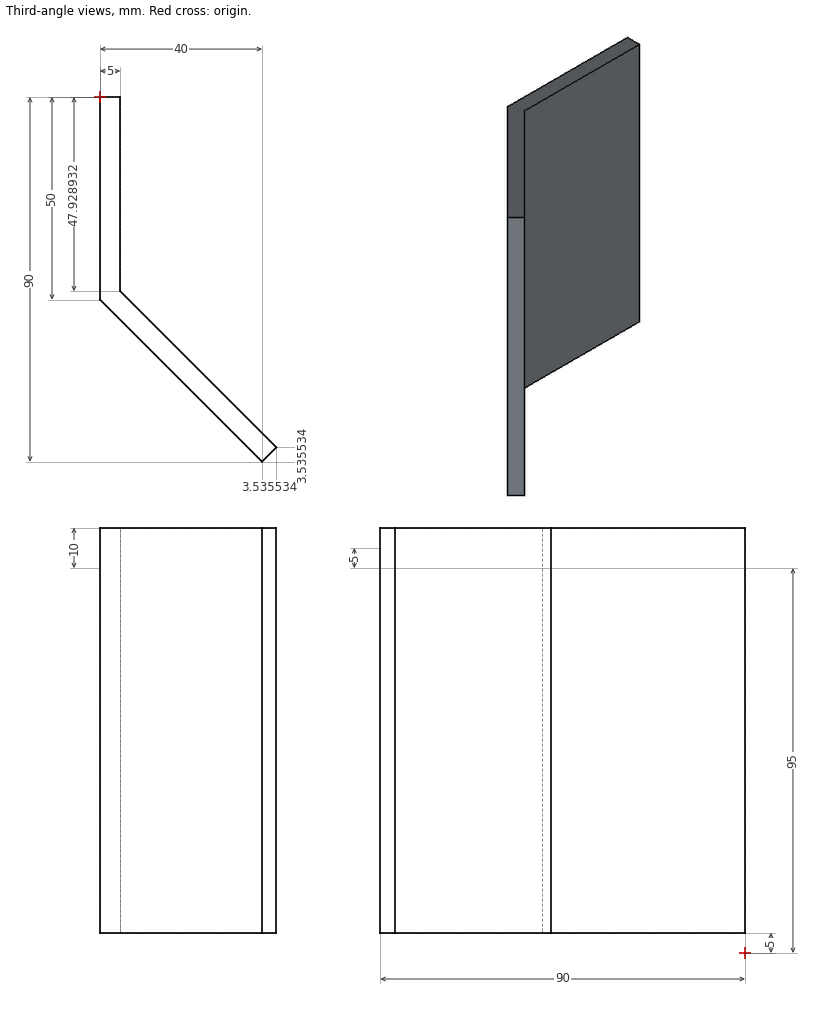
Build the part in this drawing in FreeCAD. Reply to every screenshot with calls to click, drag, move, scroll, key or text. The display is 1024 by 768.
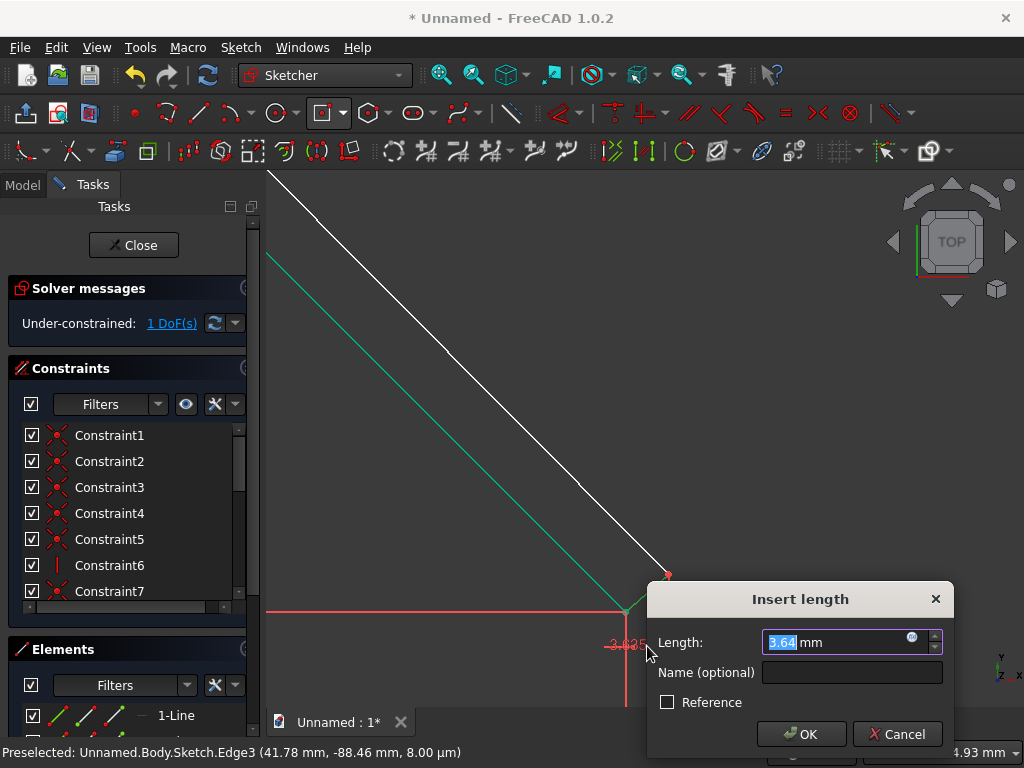
text(3.535534)
key(Return)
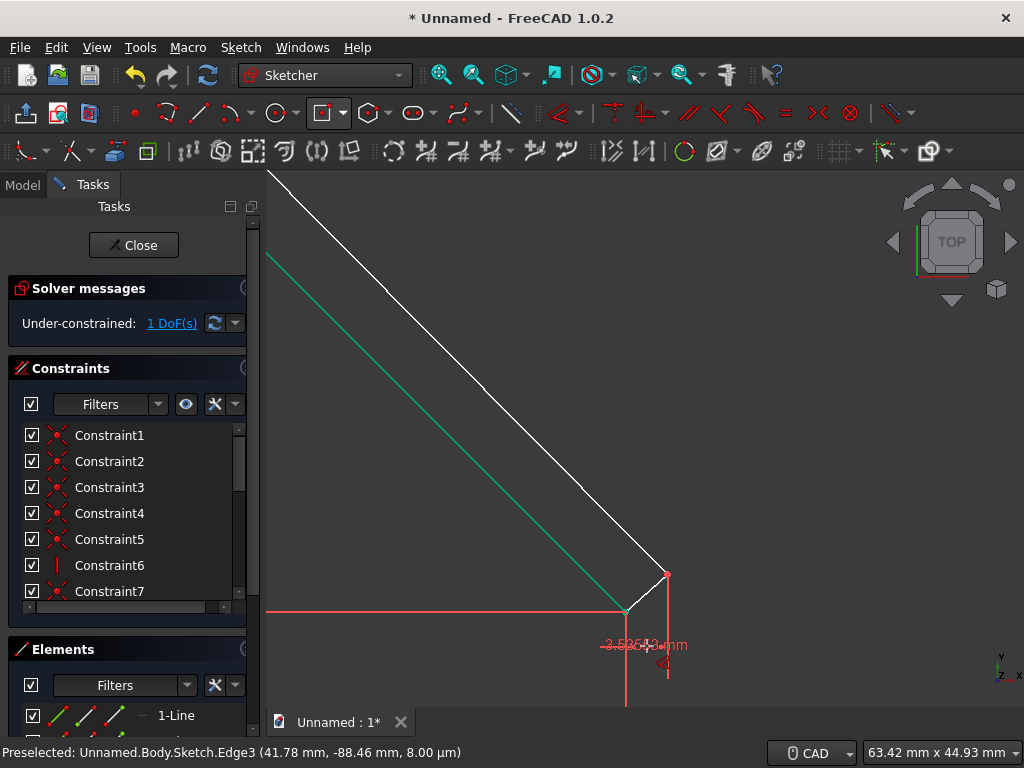
click(638, 601)
click(702, 593)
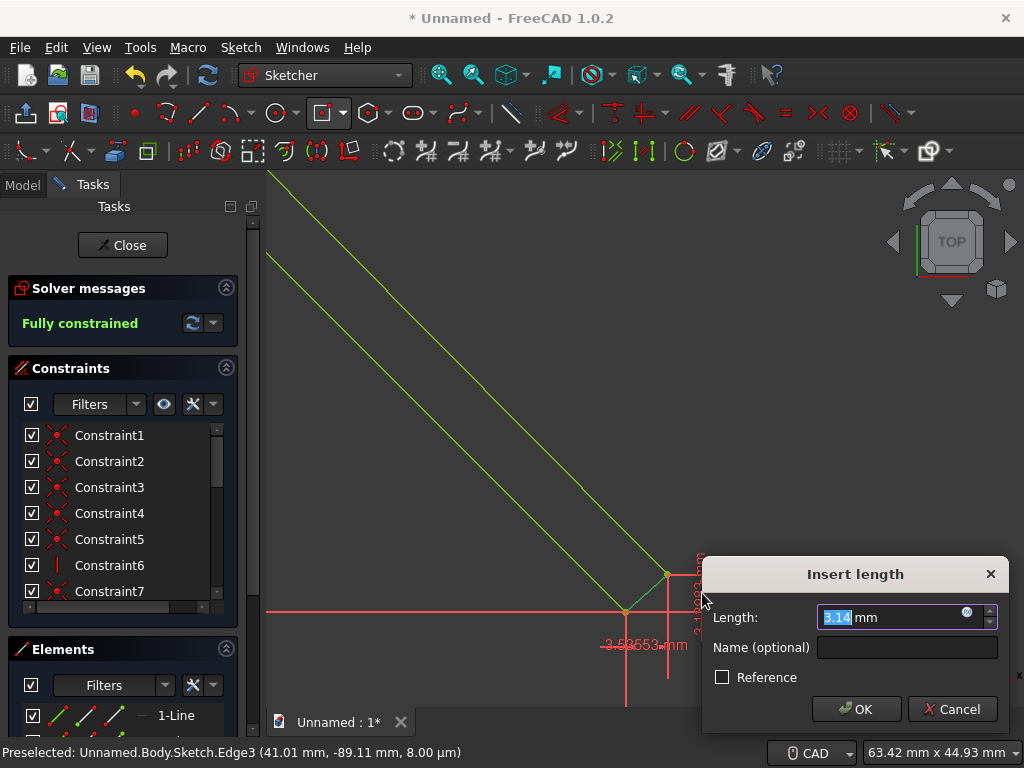
text(3.535534)
key(Return)
key(Escape)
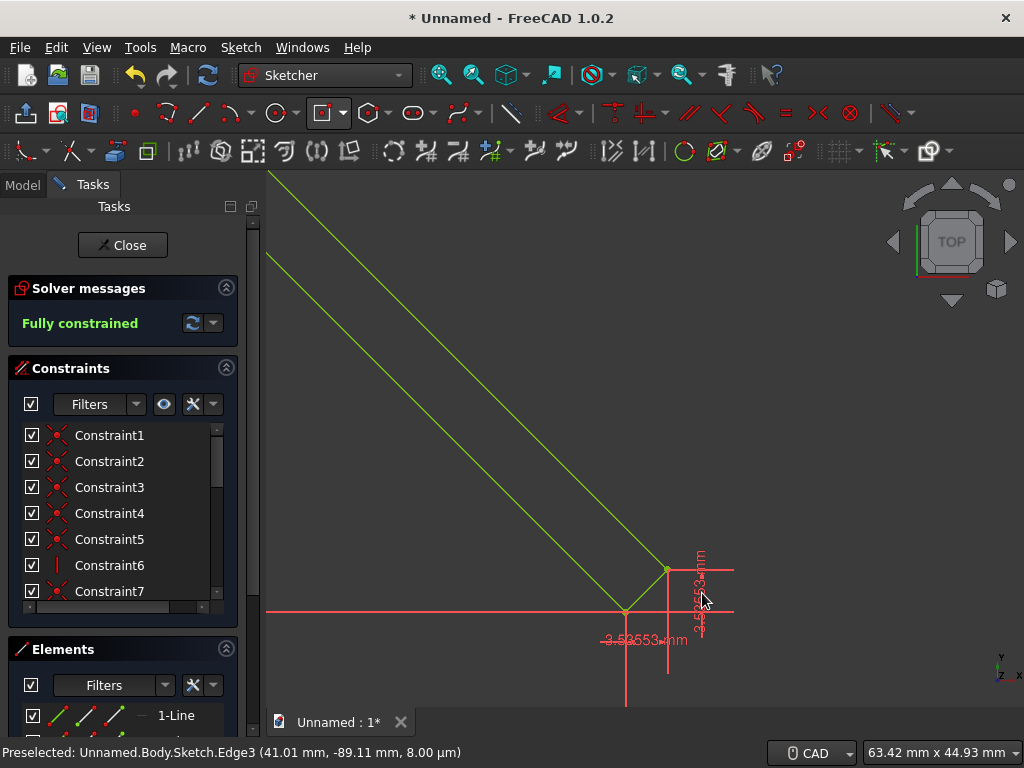
click(123, 245)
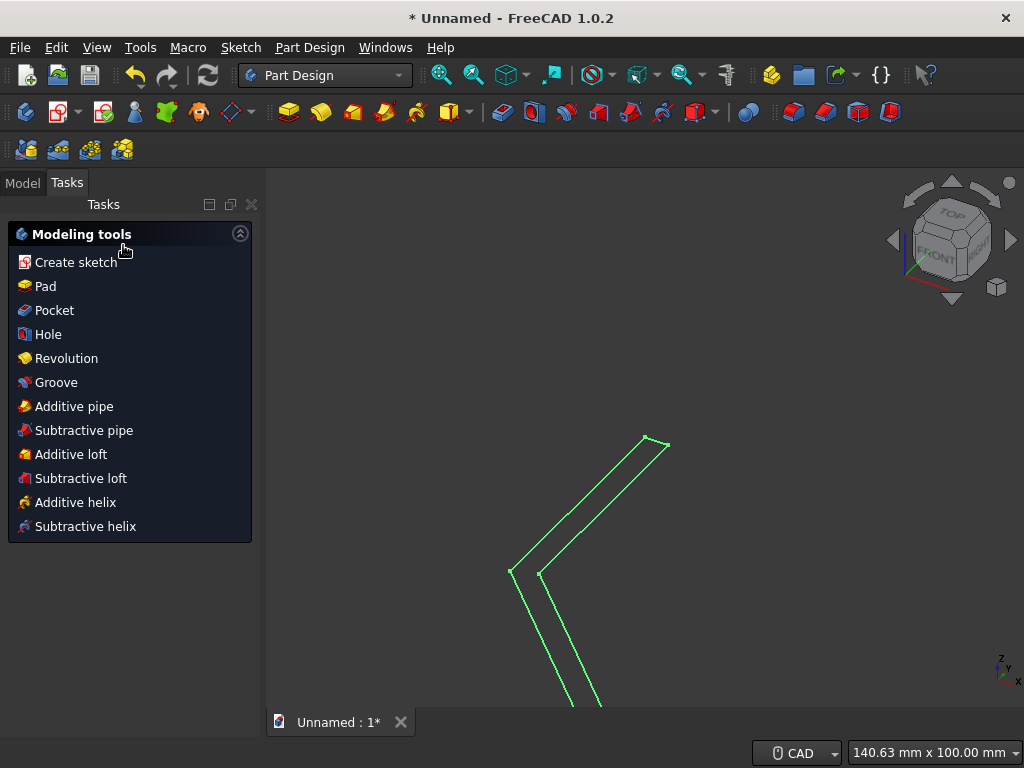
click(290, 112)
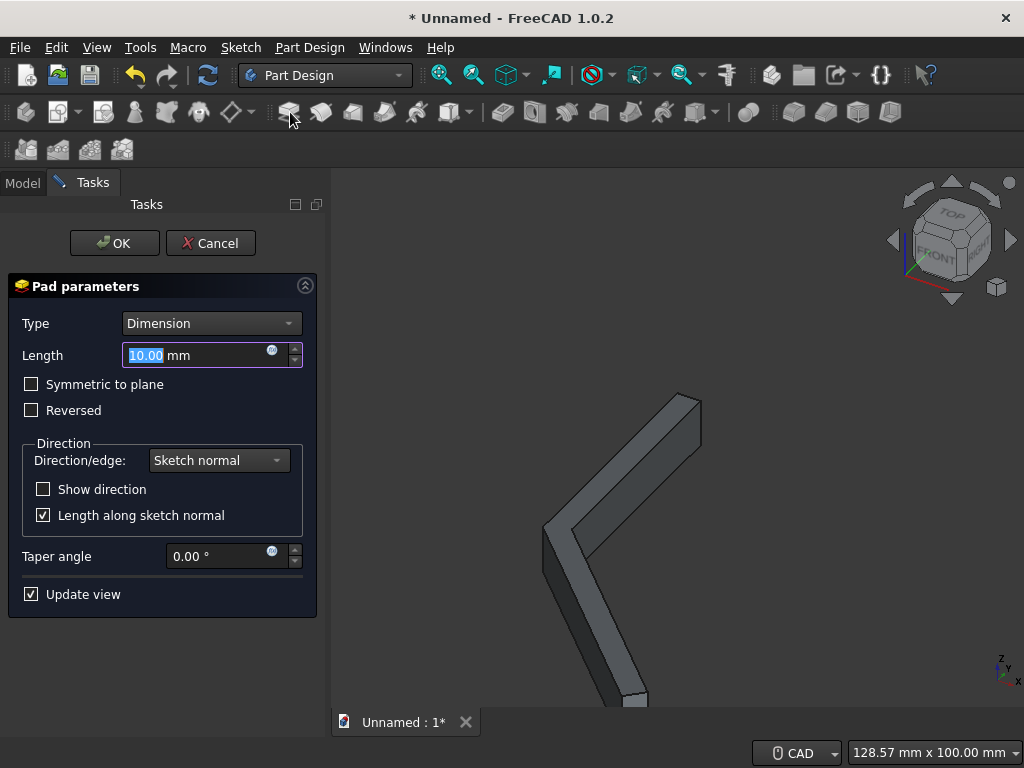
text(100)
key(Tab)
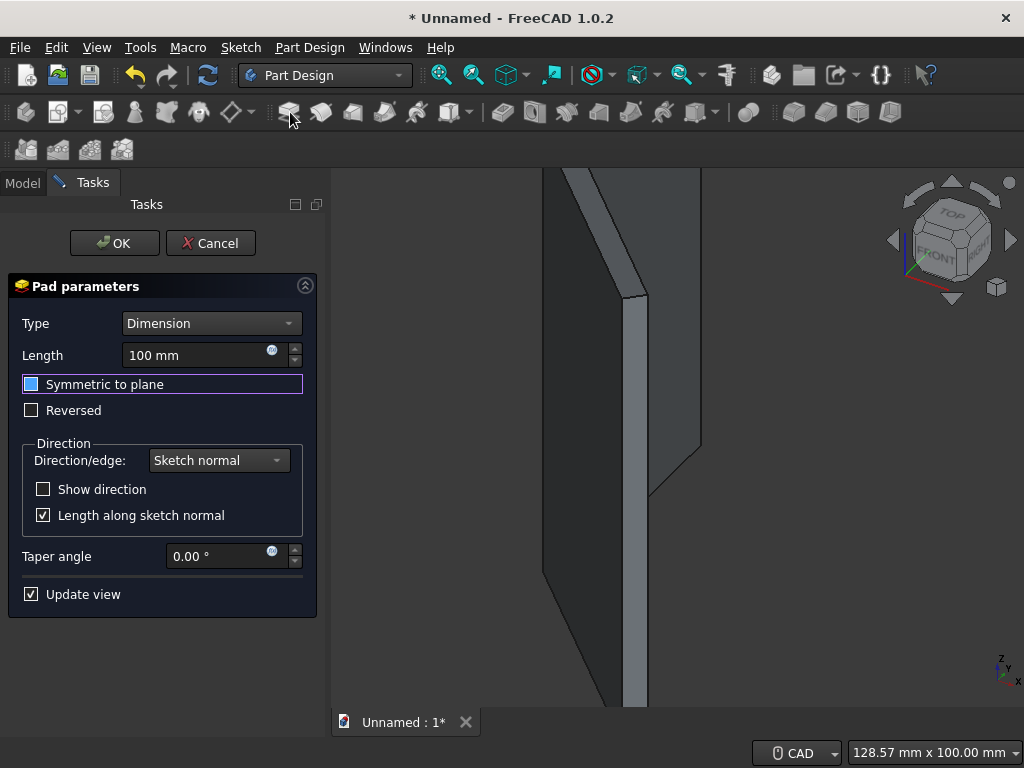
click(115, 243)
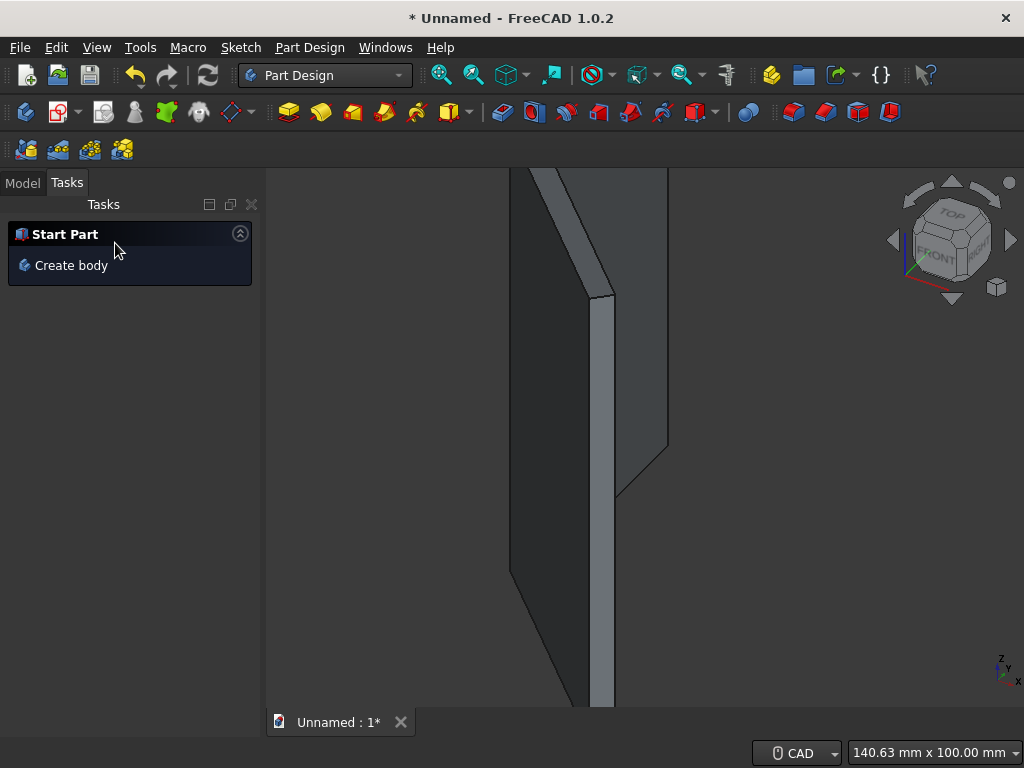
click(442, 76)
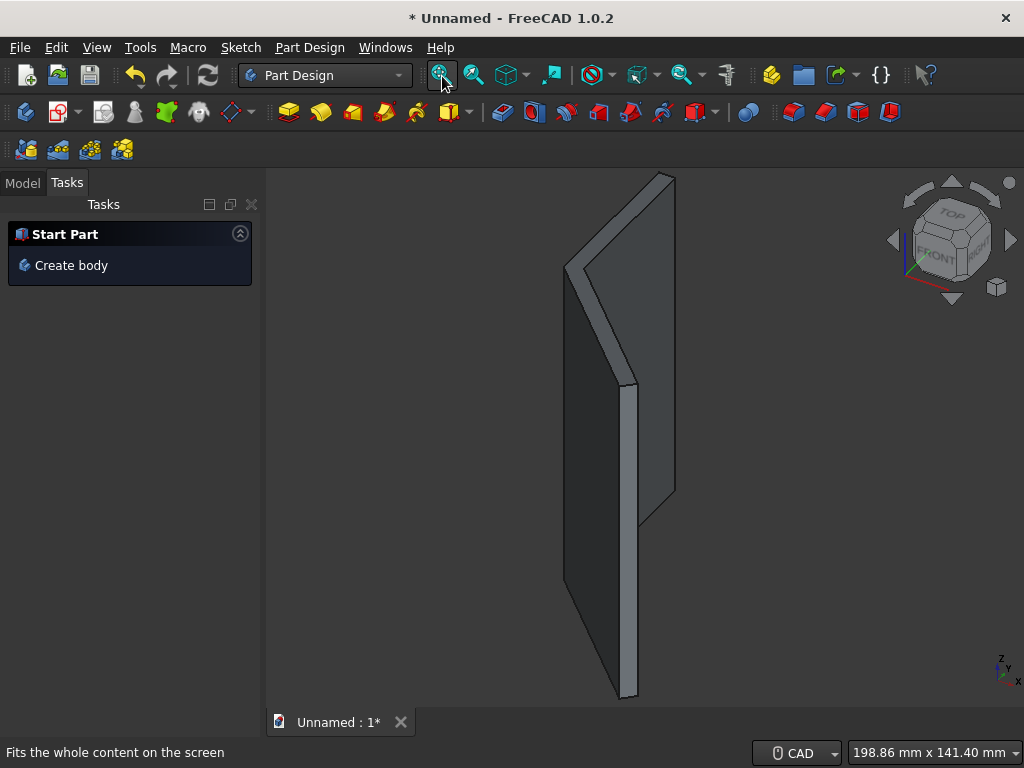
click(630, 334)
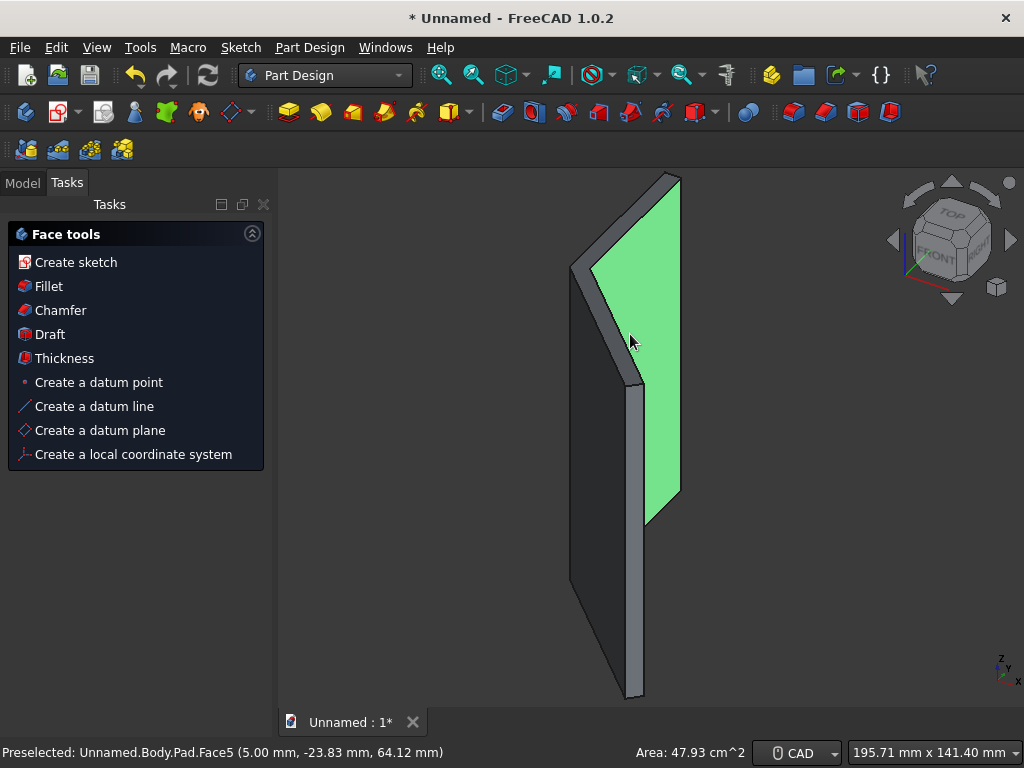
click(58, 112)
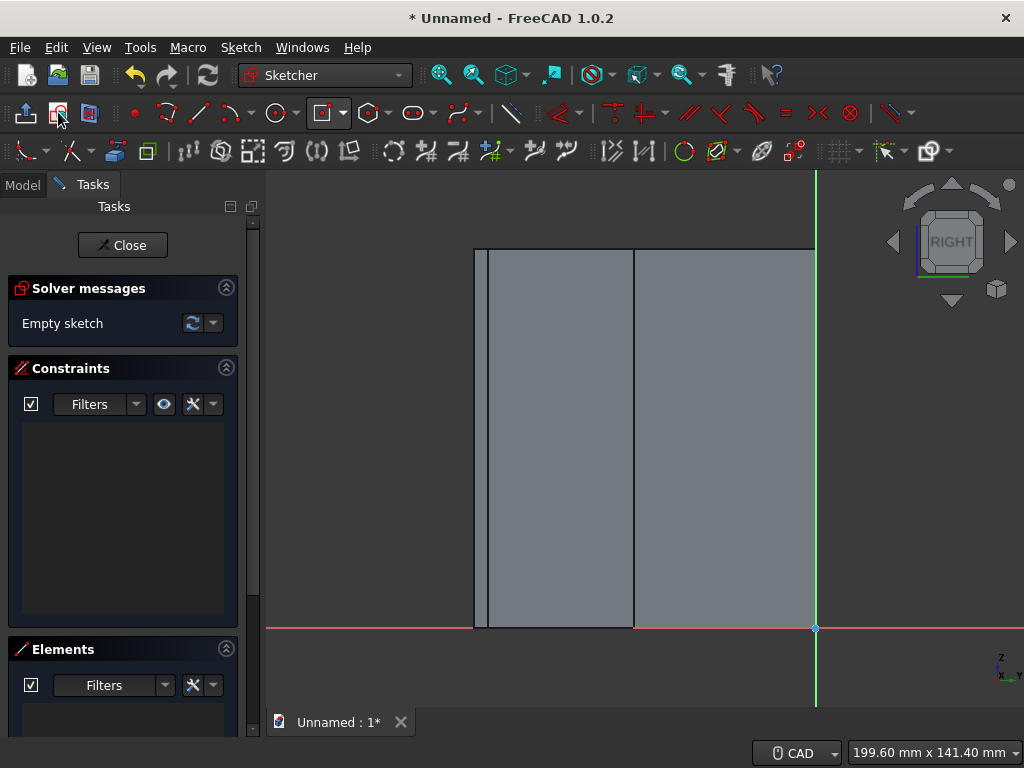
click(90, 114)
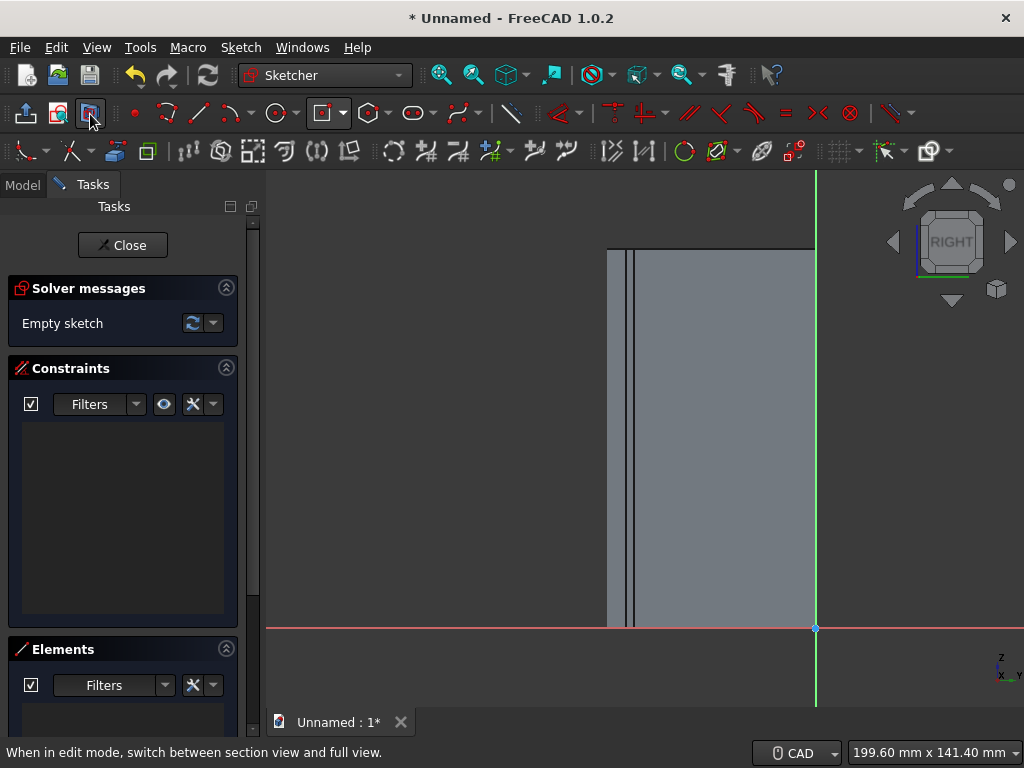
click(346, 114)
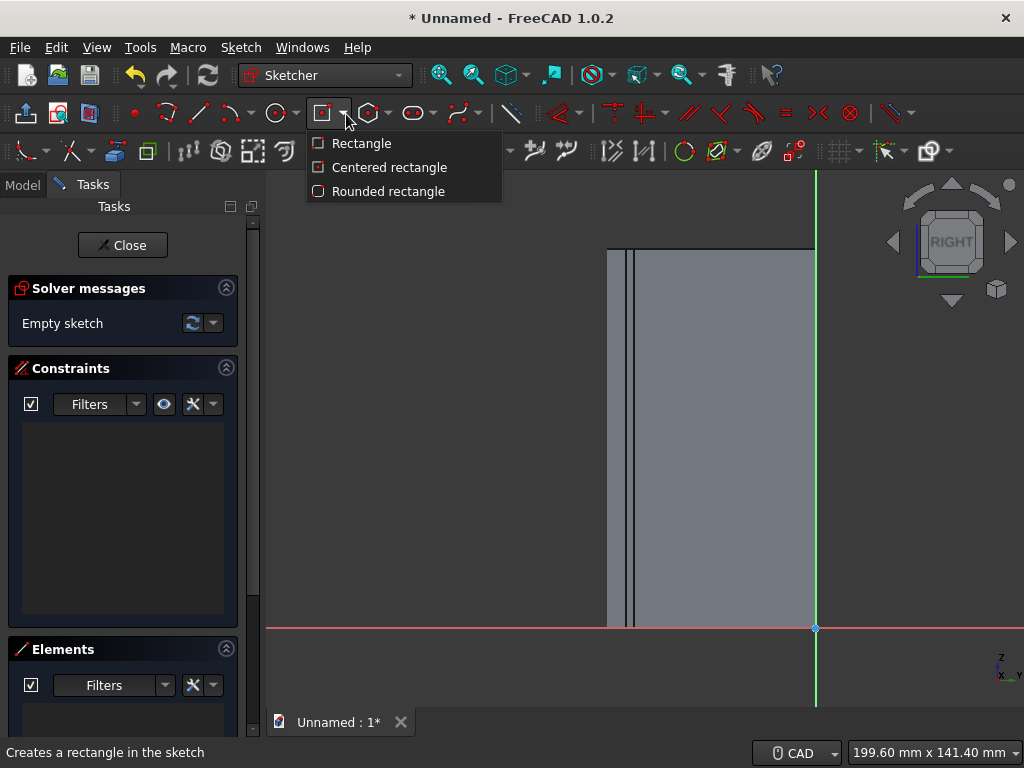
click(404, 143)